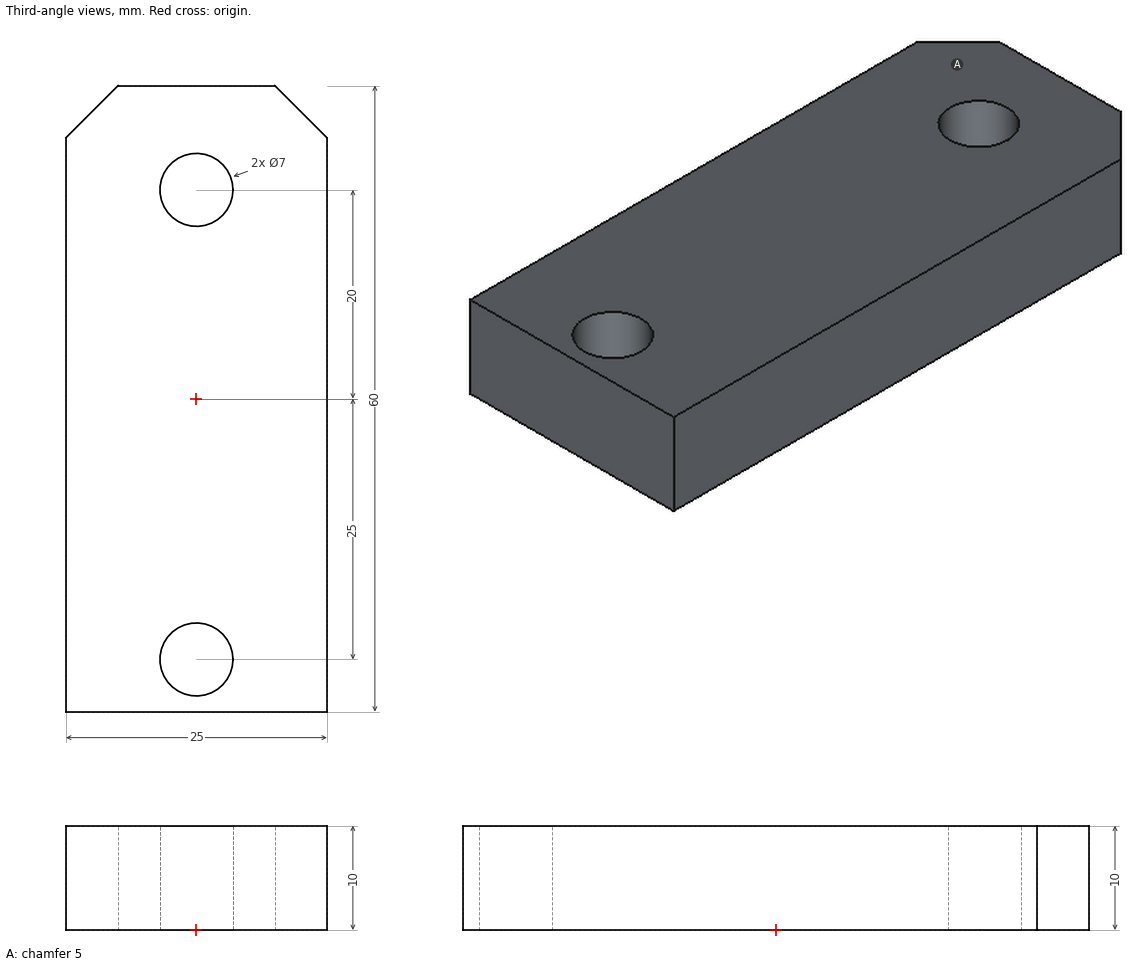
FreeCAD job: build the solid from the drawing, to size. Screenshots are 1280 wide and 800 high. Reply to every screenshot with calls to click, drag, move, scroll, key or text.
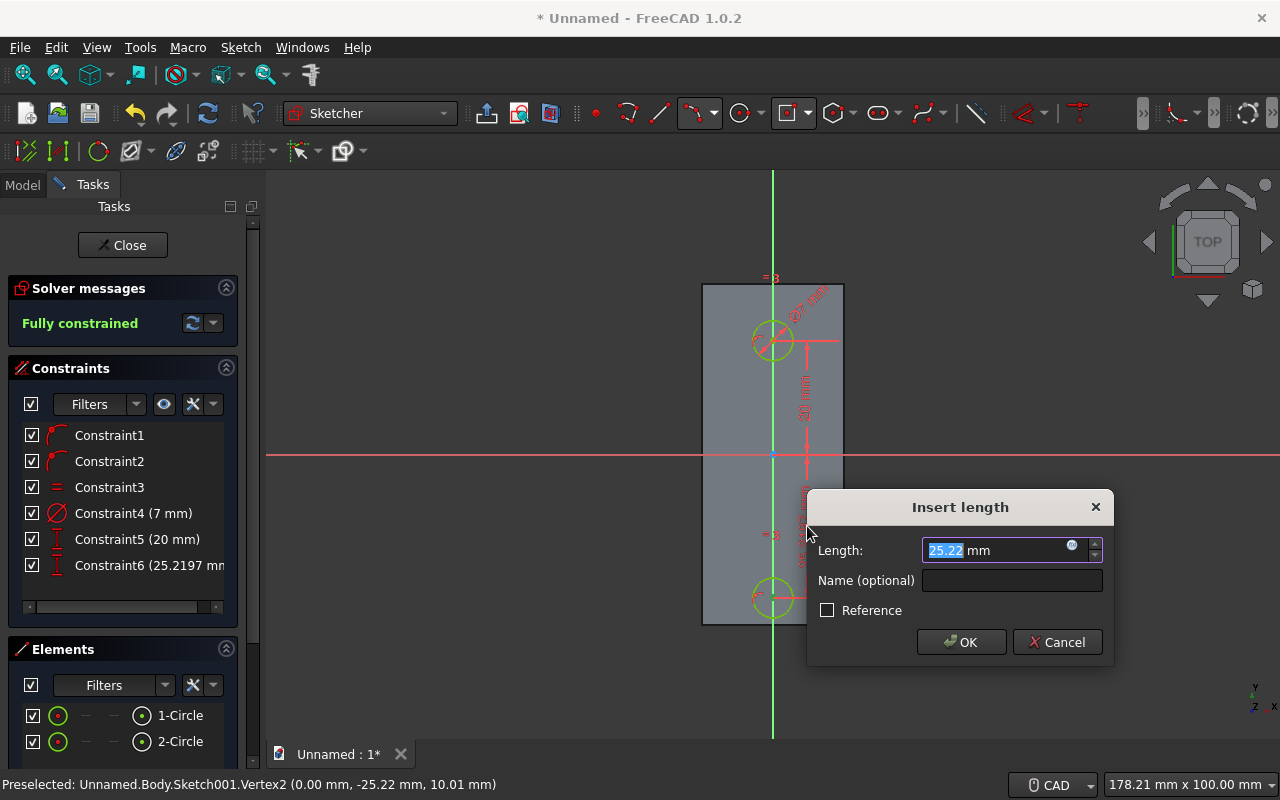
text(25)
key(Return)
key(Escape)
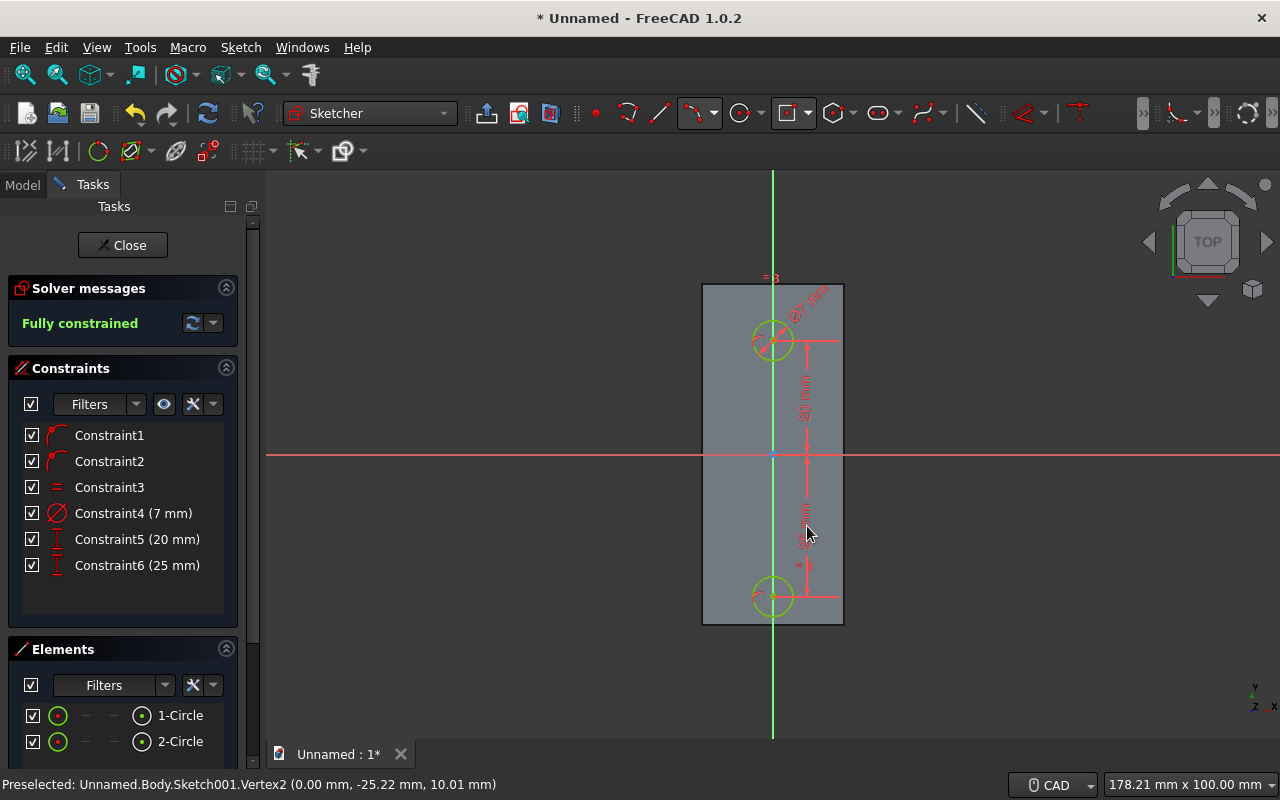
click(123, 245)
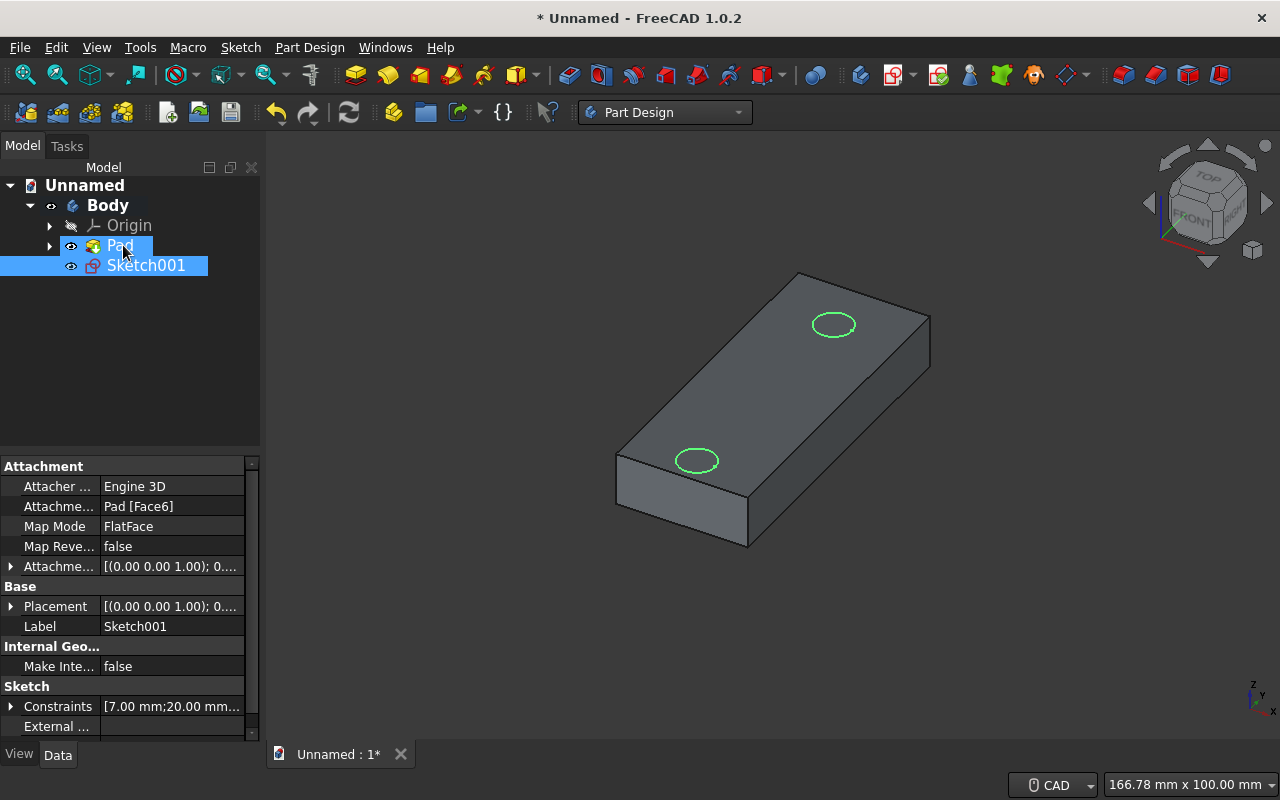
click(570, 76)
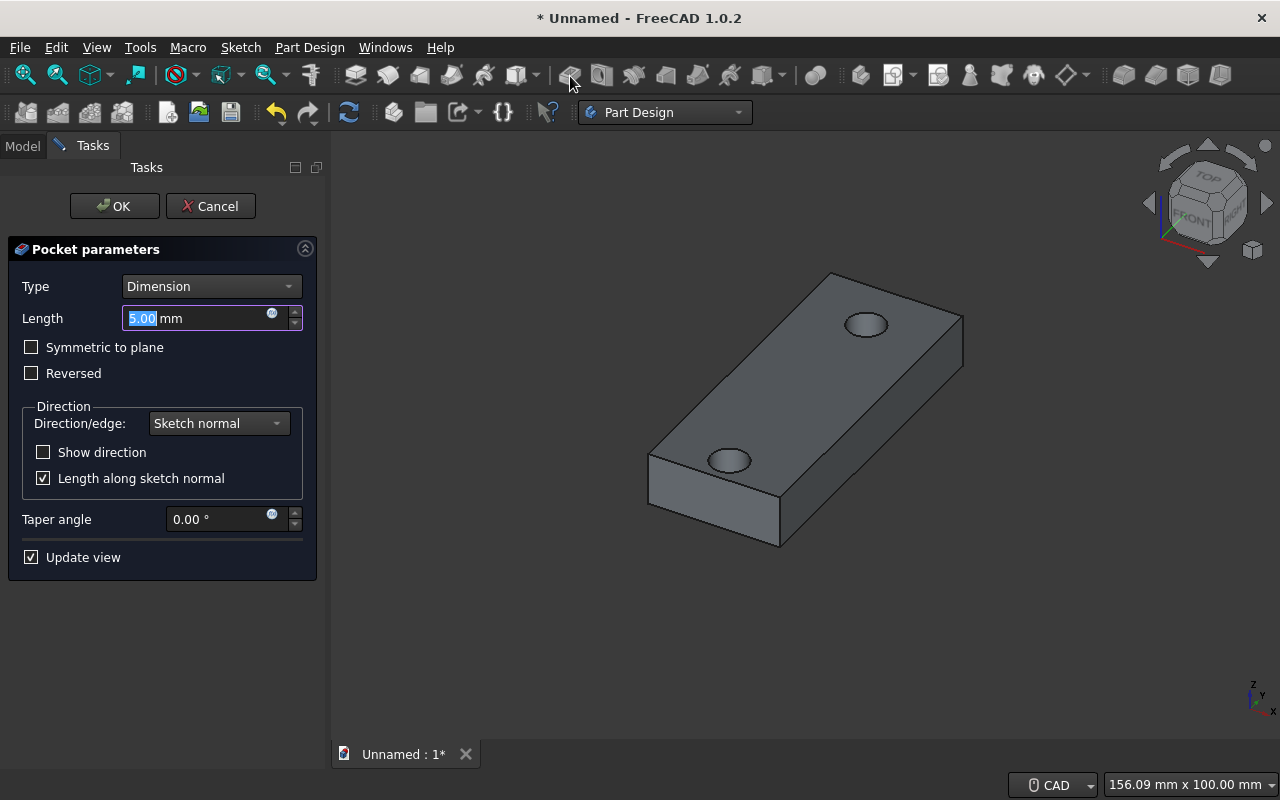
text(10)
key(Tab)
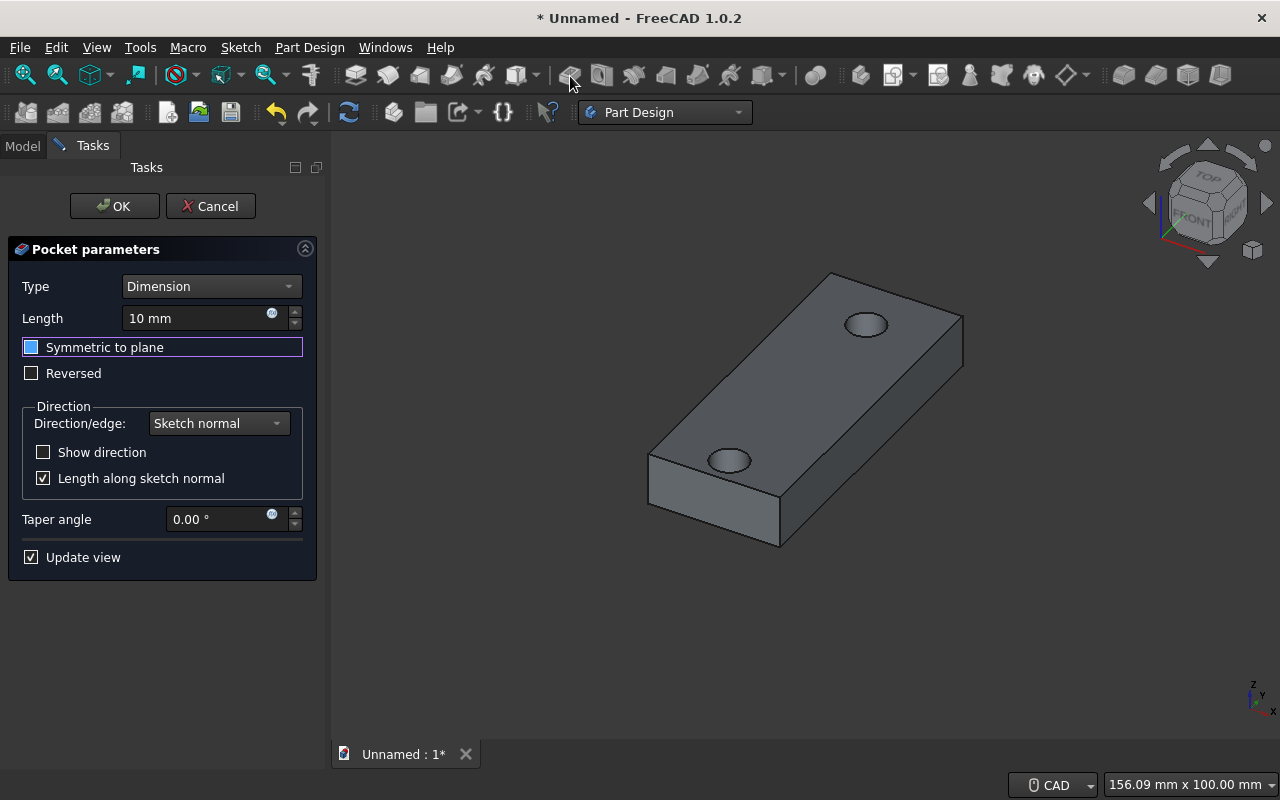
click(115, 206)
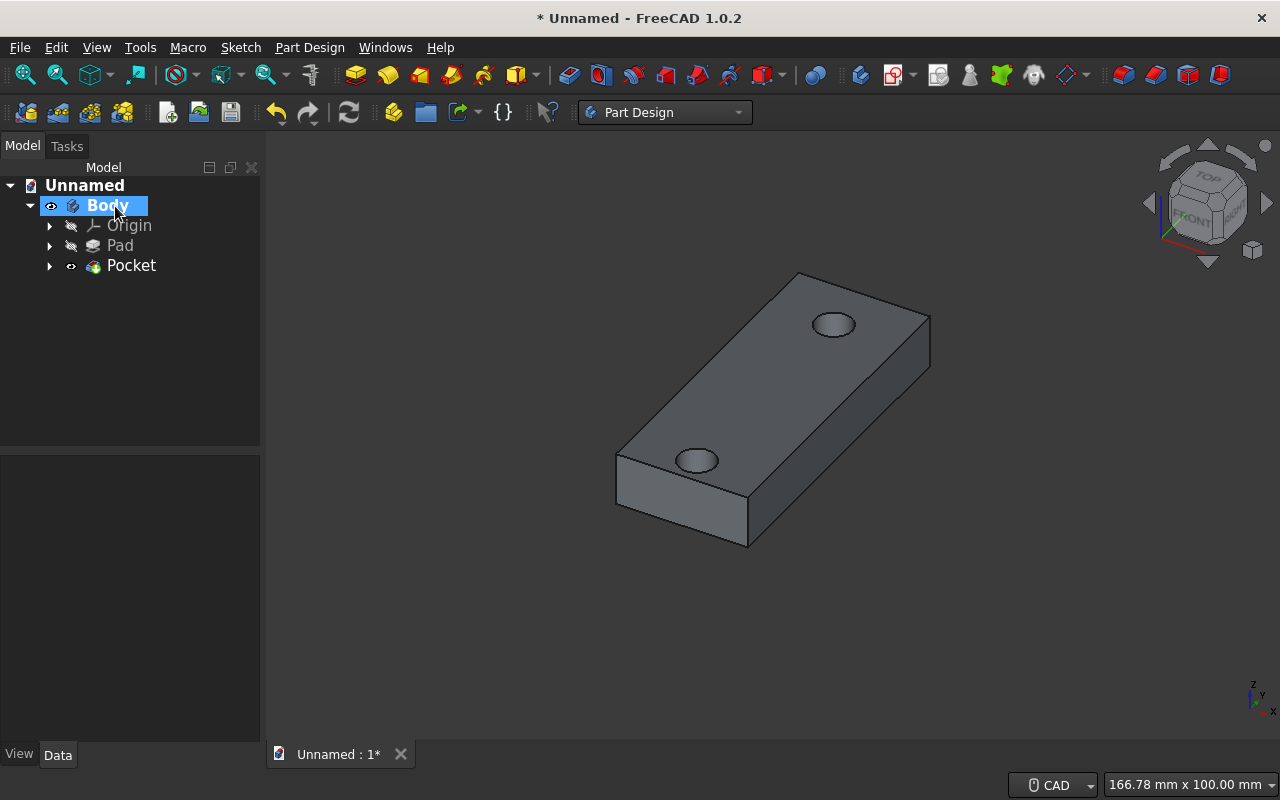
key(0)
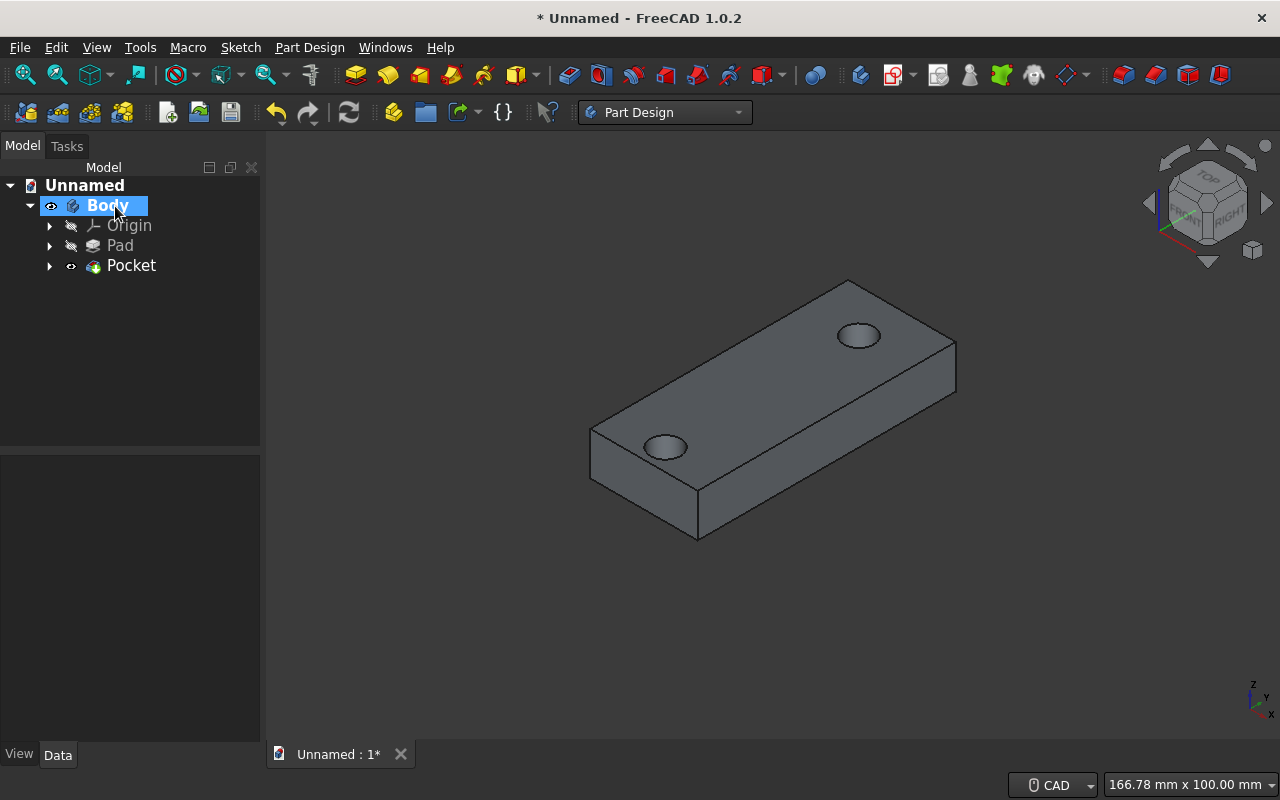
click(26, 76)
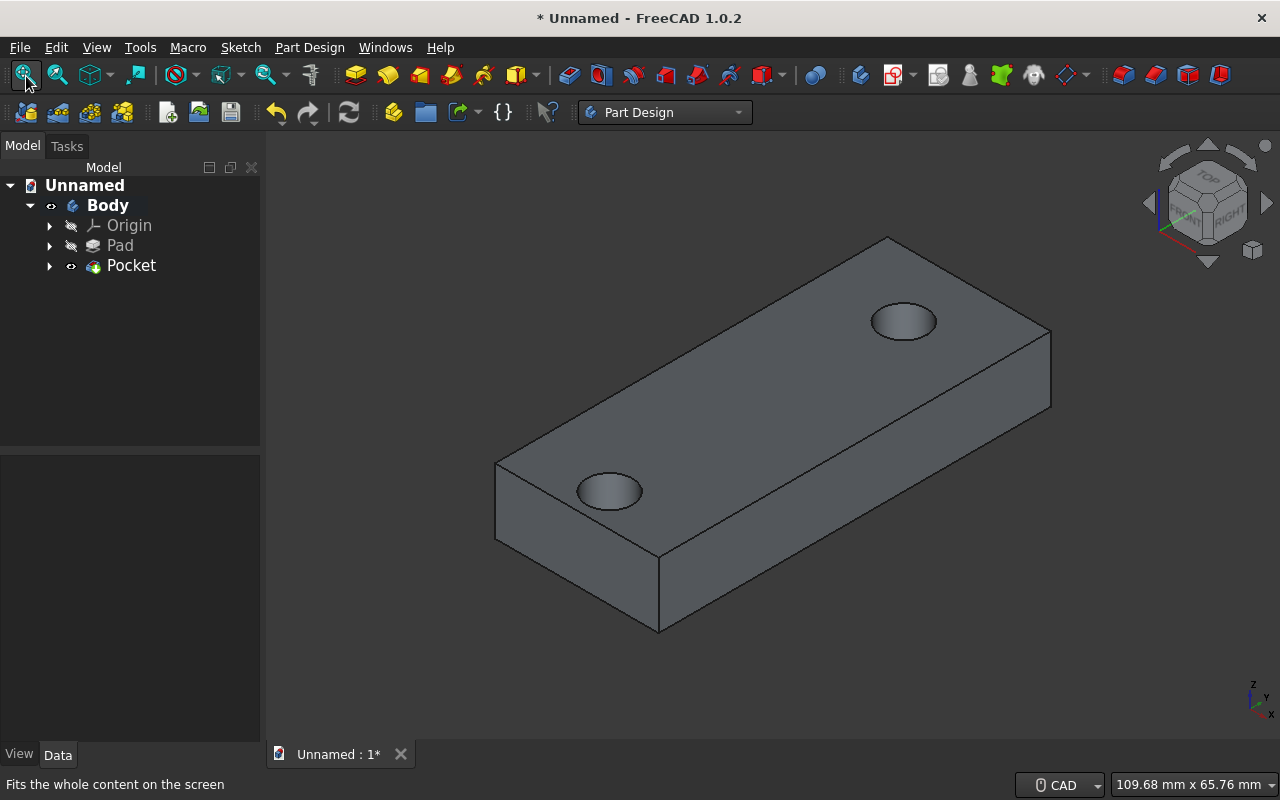
key(2)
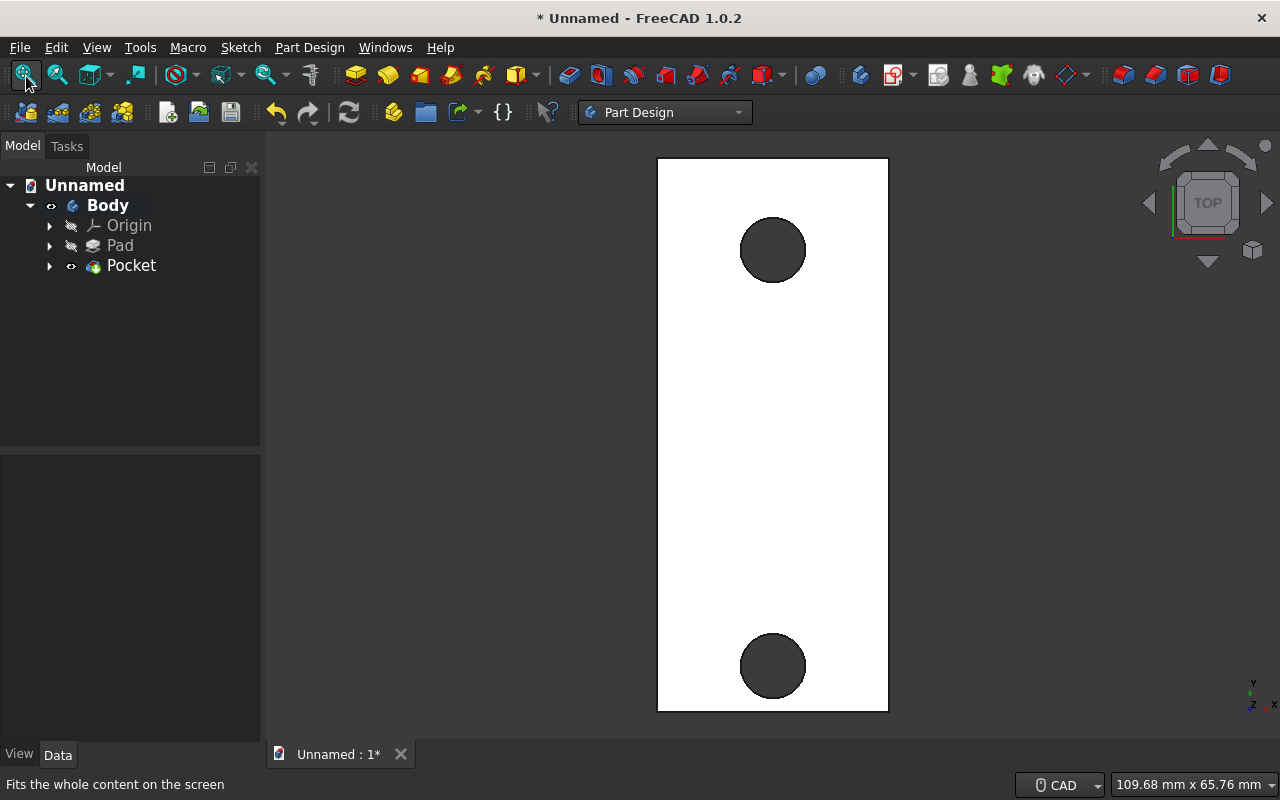
key(1)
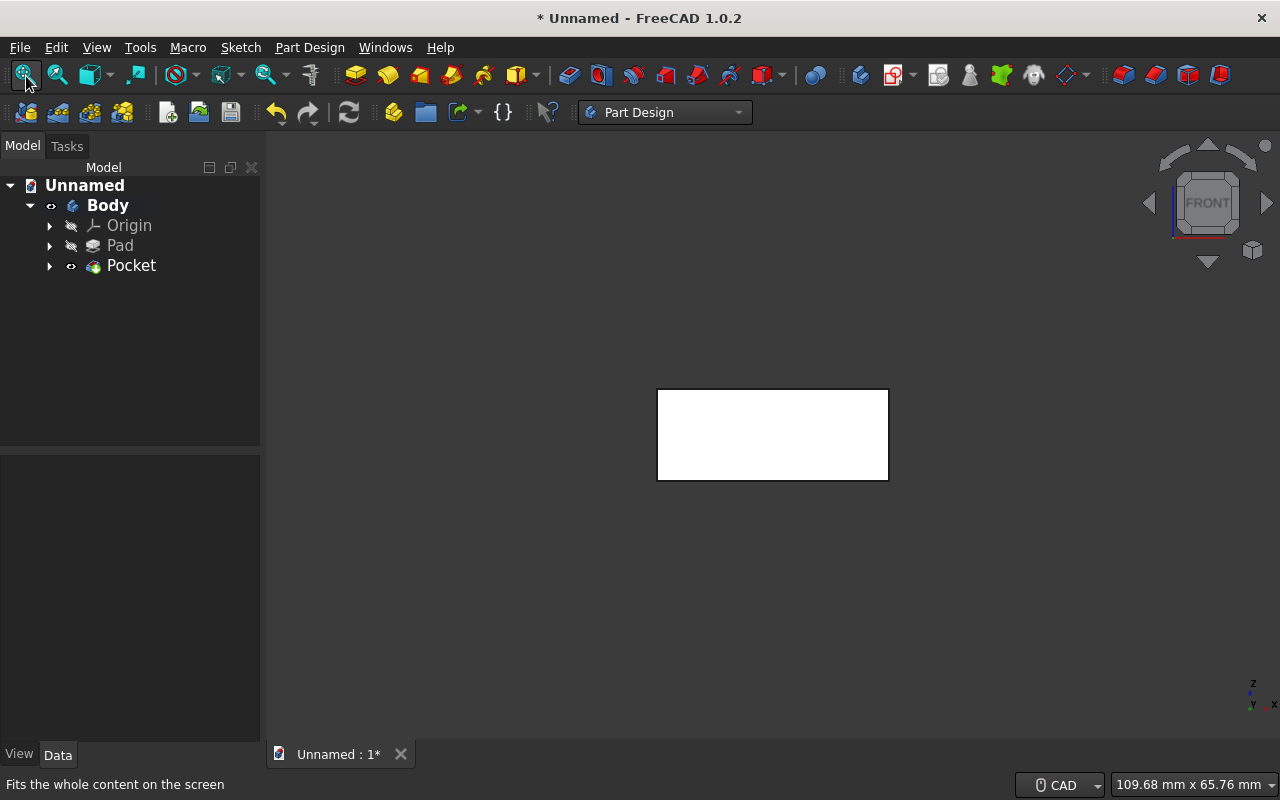
click(26, 76)